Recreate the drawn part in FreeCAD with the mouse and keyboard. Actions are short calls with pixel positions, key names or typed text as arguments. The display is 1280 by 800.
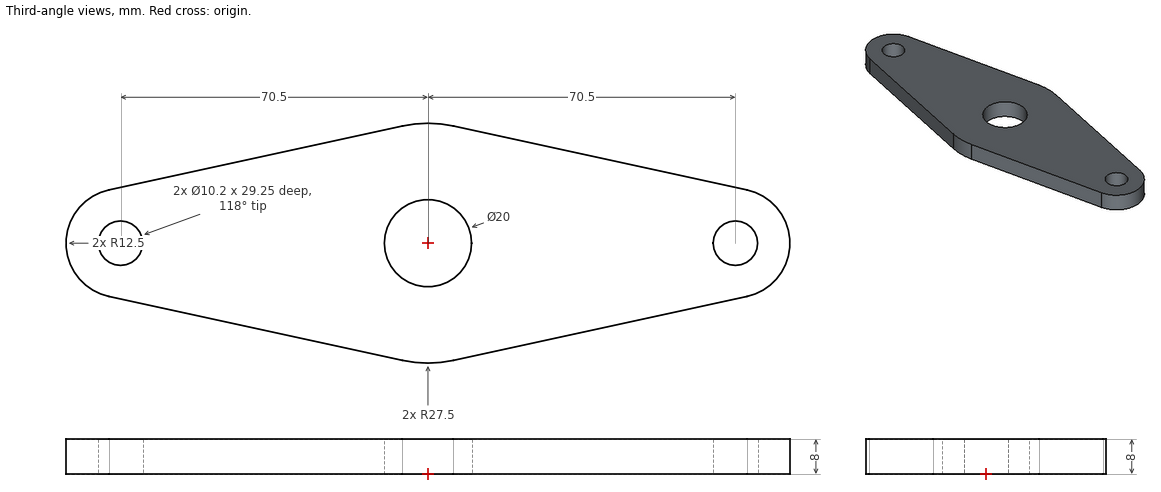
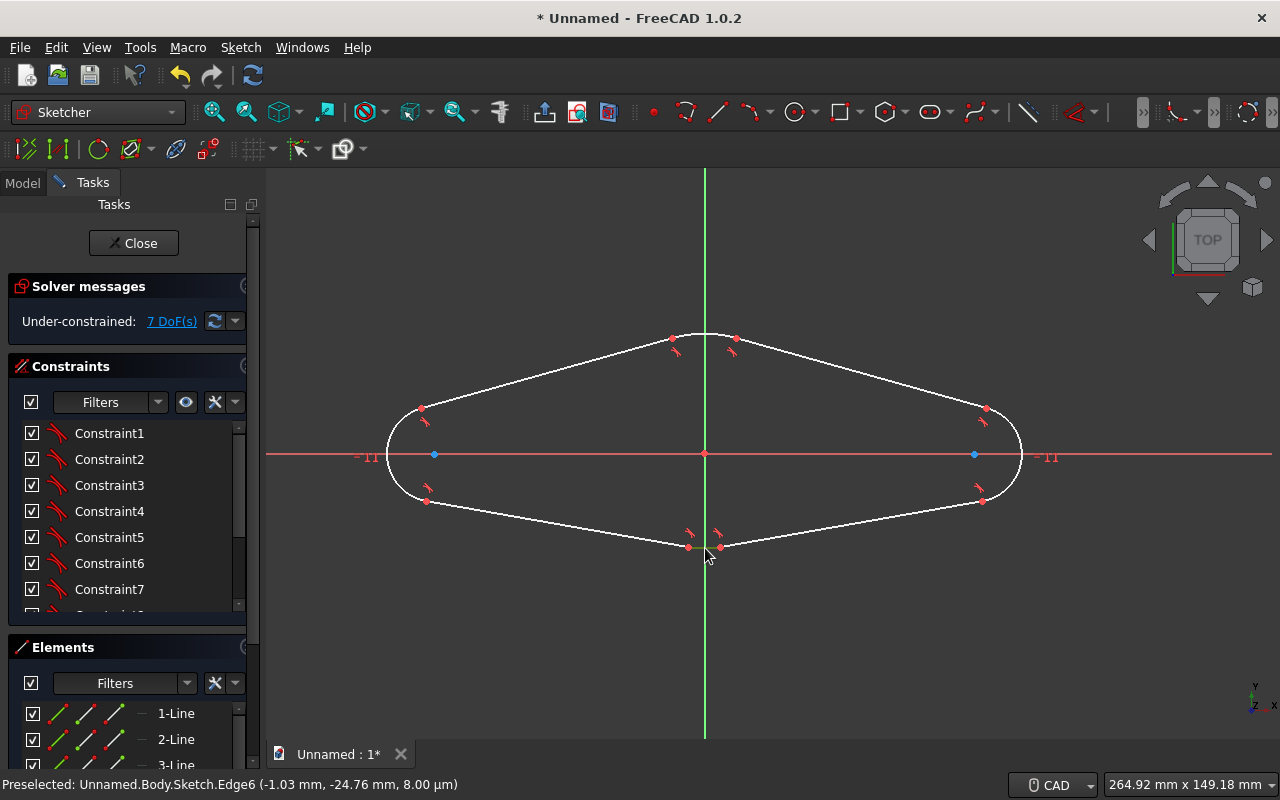
click(718, 334)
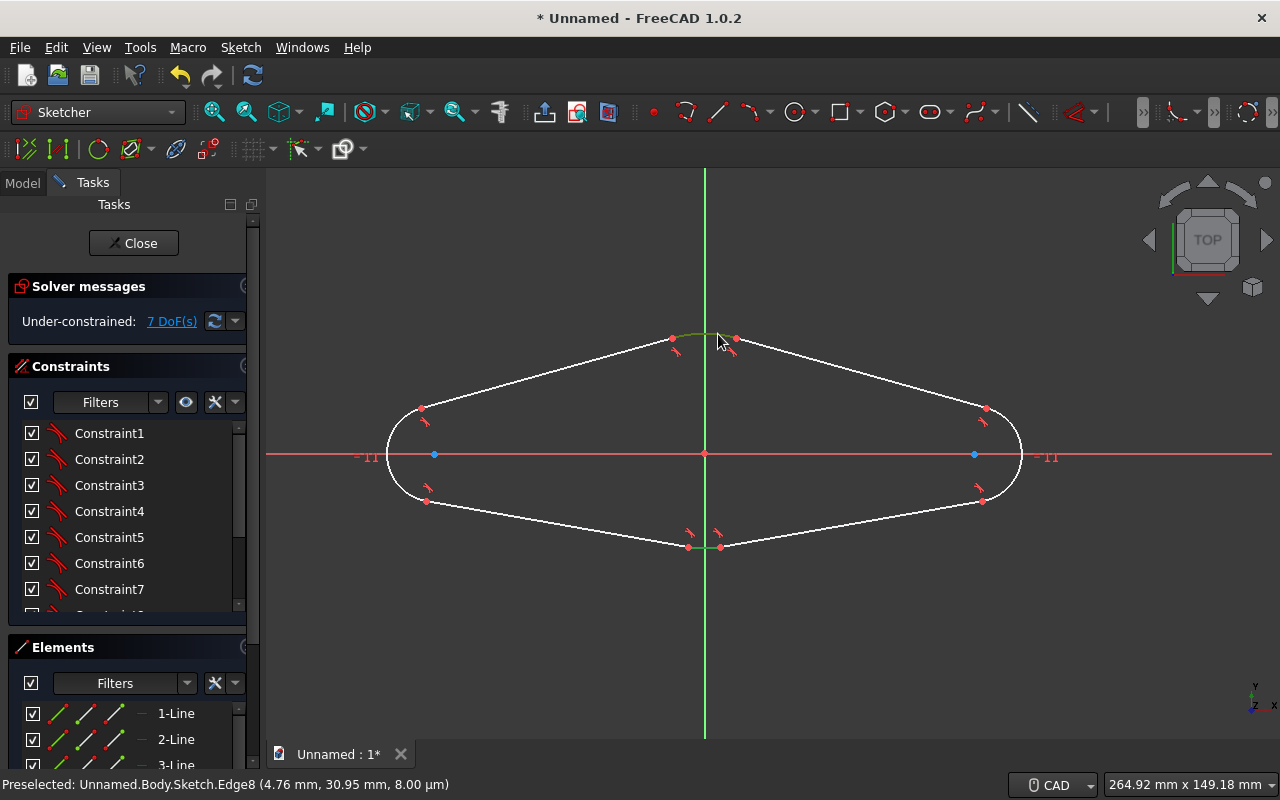
key(e)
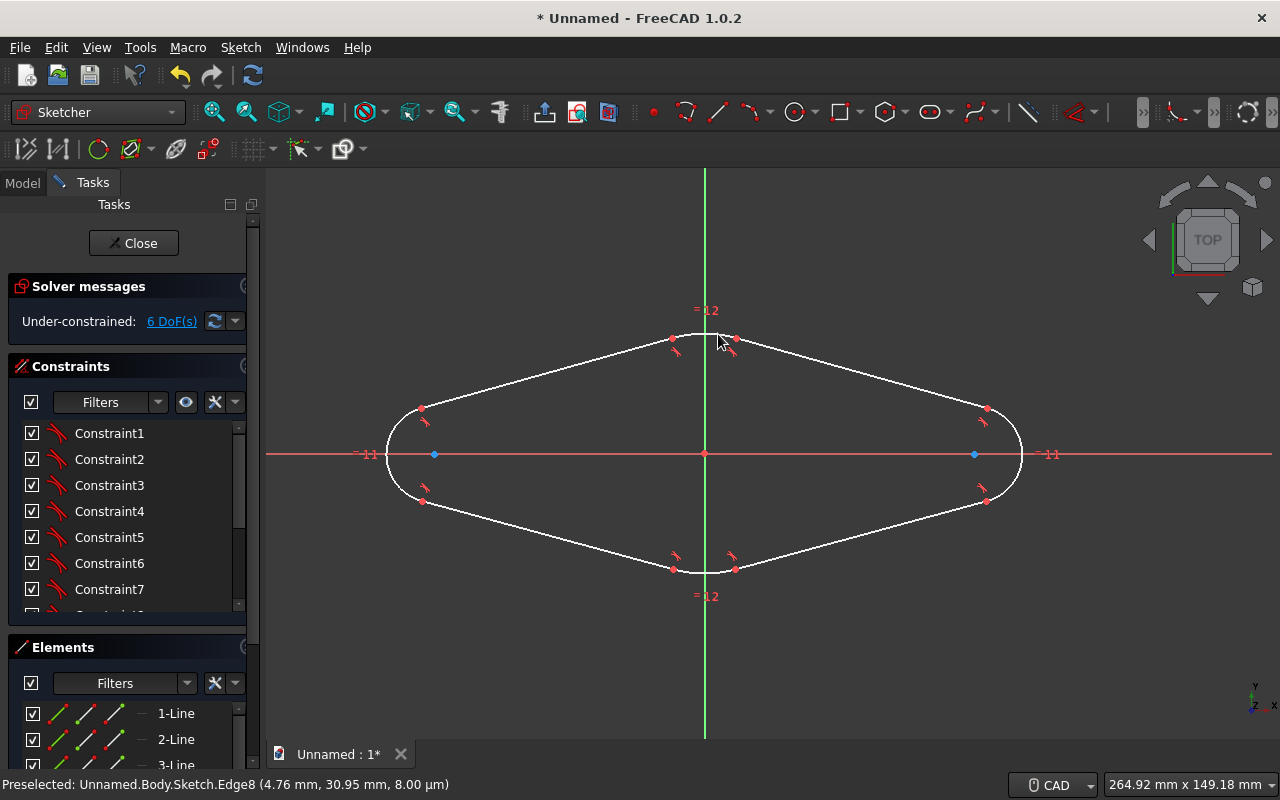
click(435, 455)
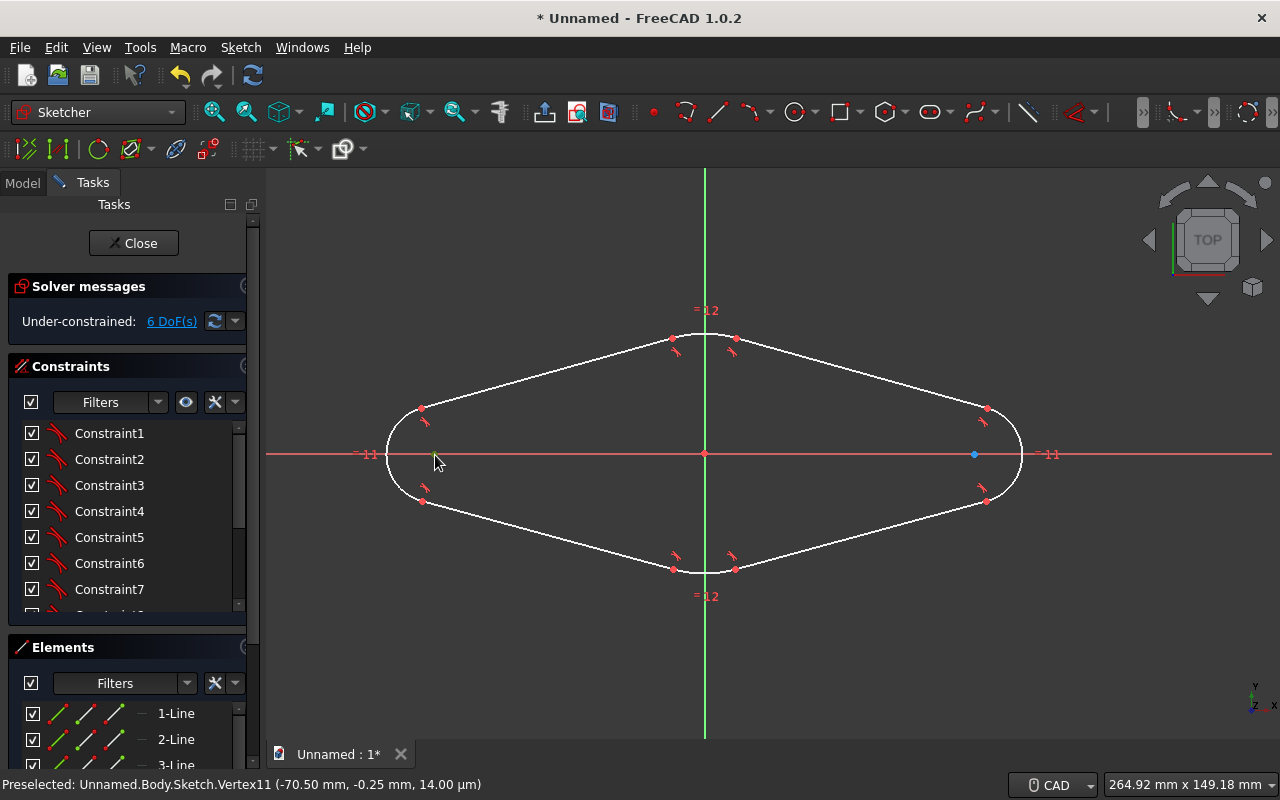
click(470, 454)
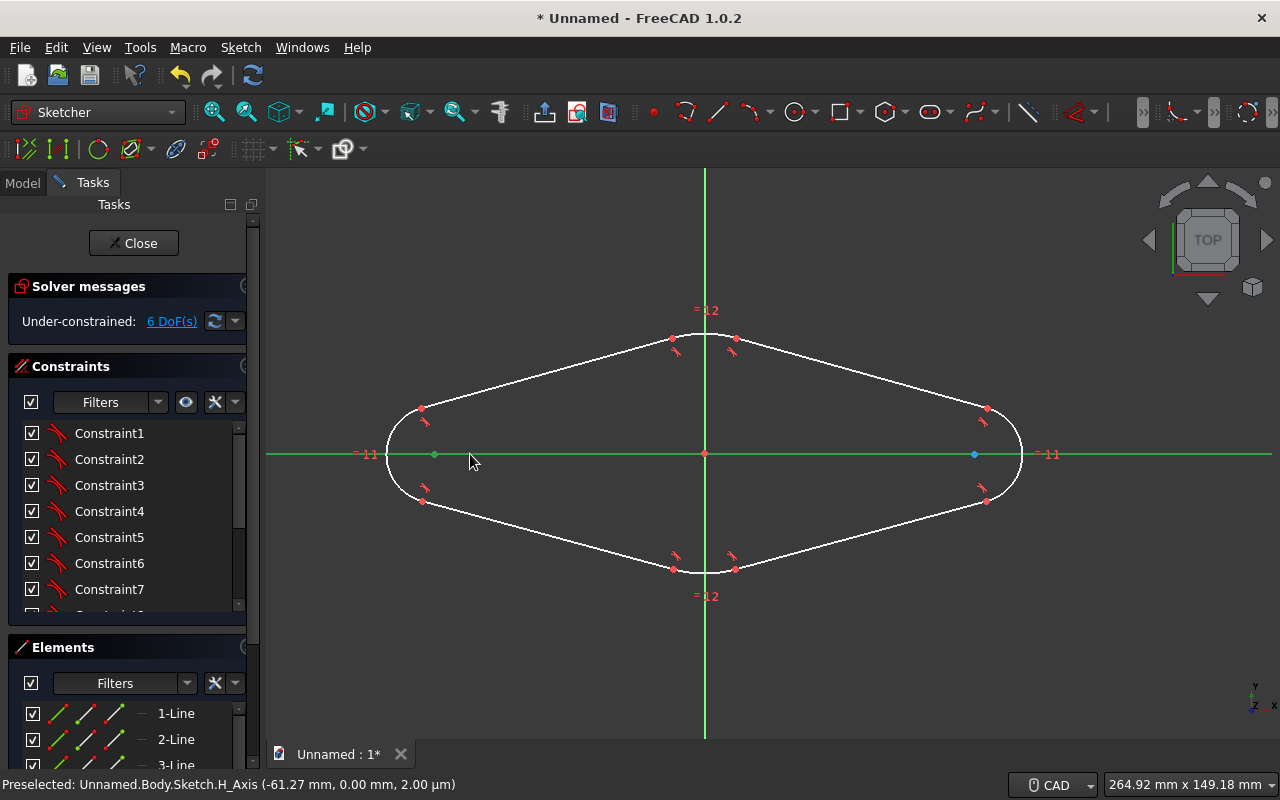
key(c)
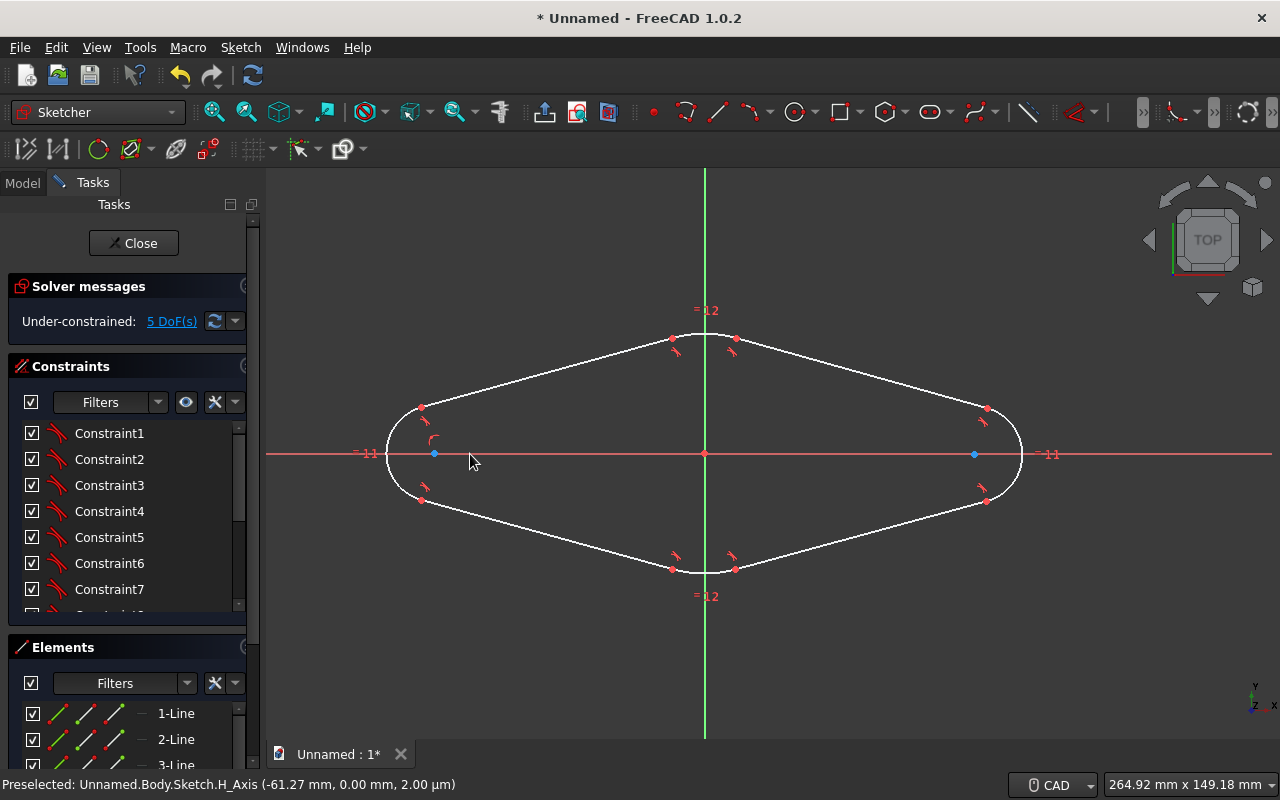
click(974, 455)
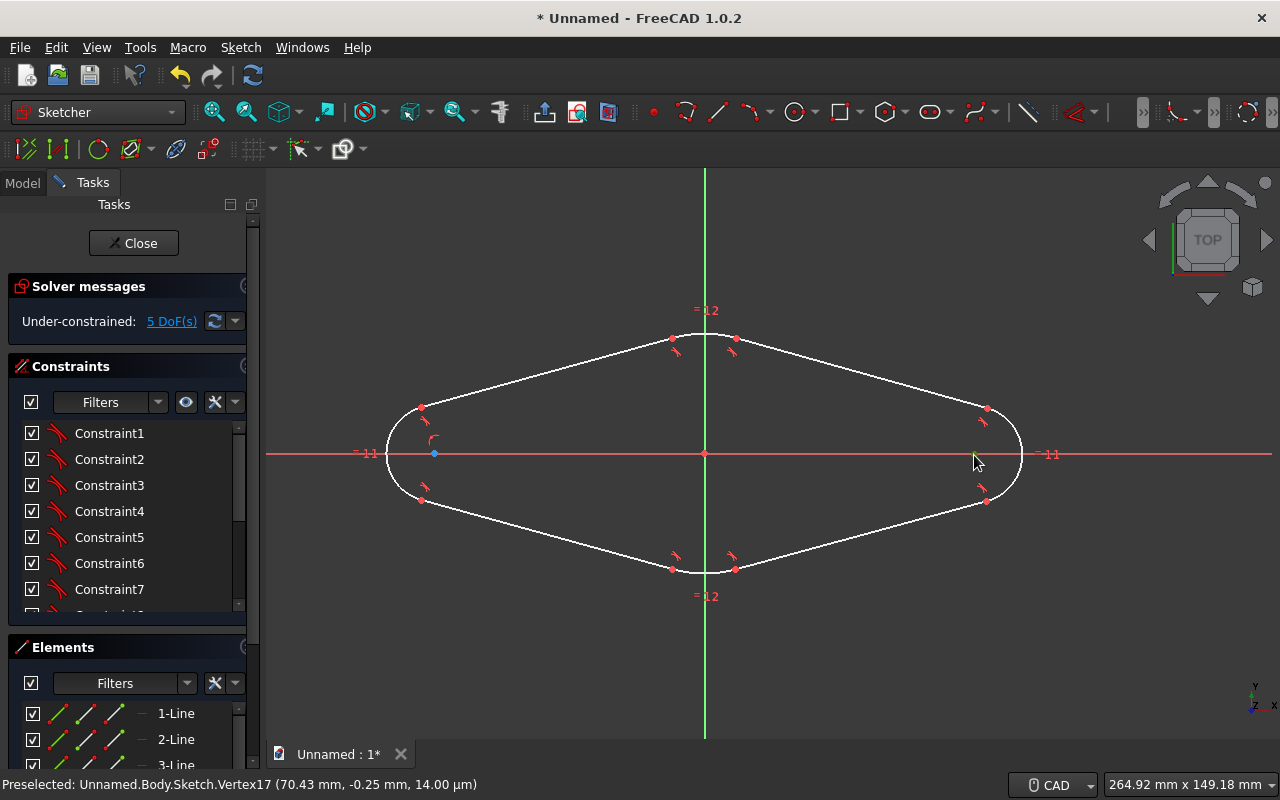
click(470, 454)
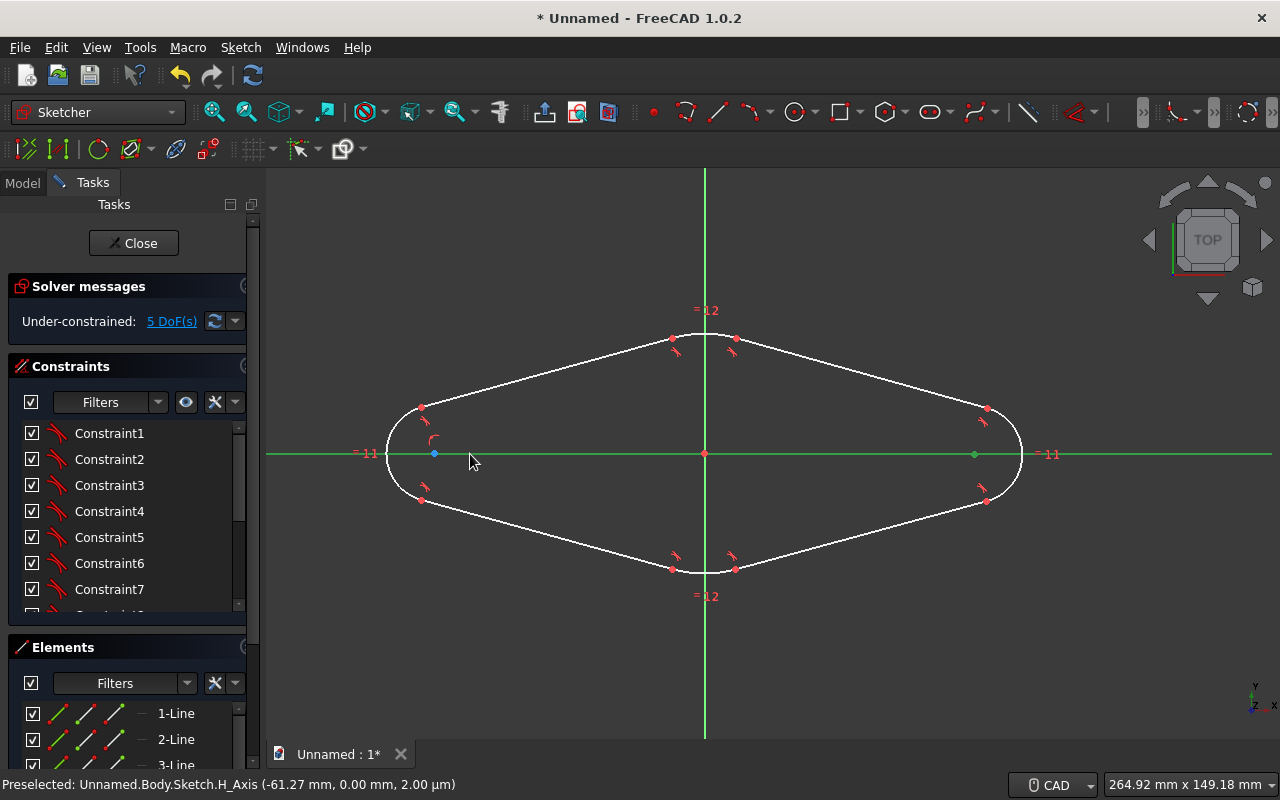
key(c)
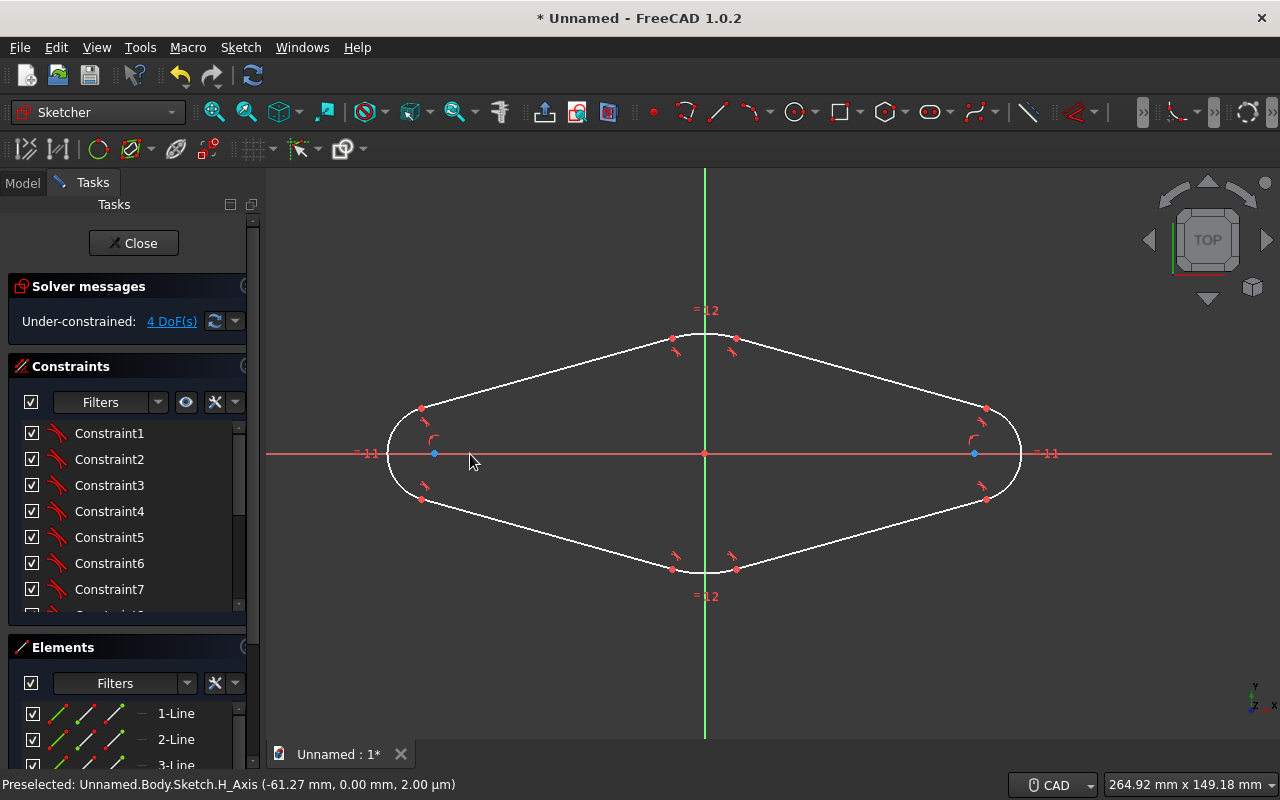
click(394, 430)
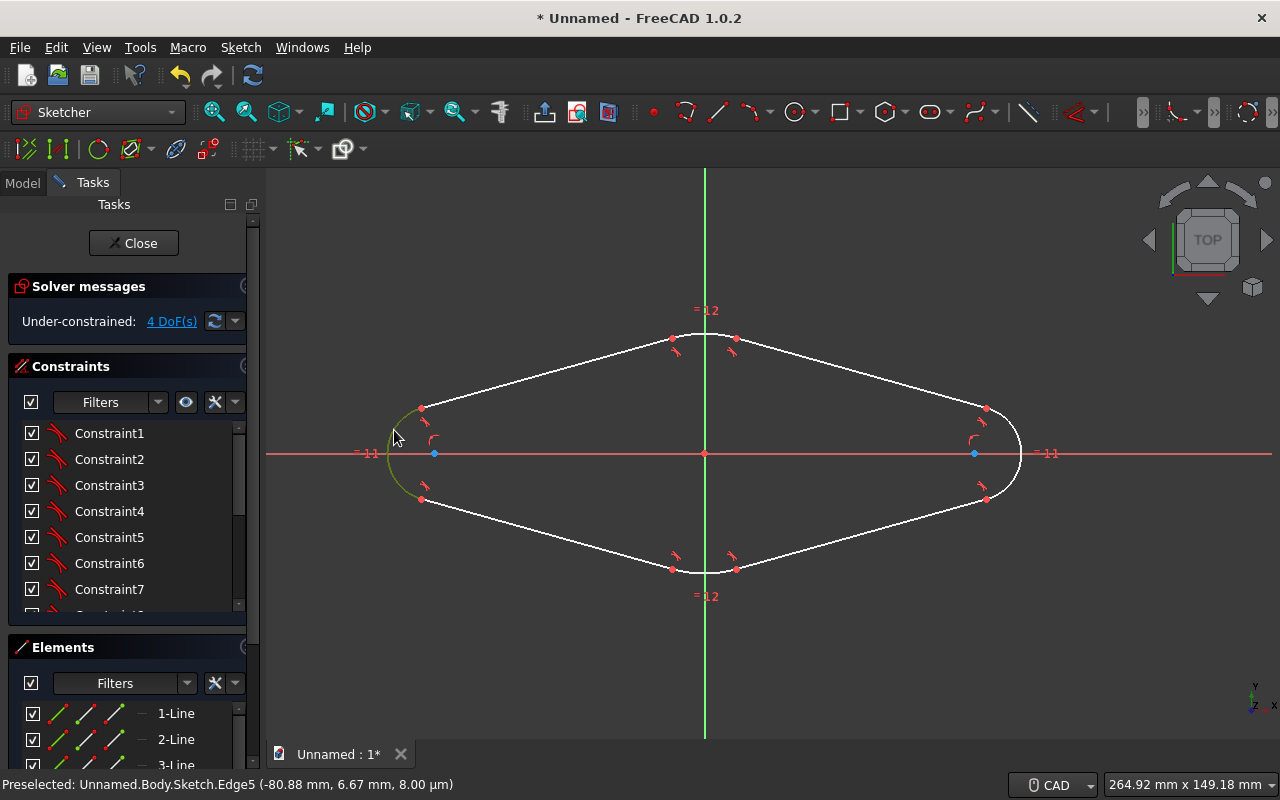
key(k)
key(r)